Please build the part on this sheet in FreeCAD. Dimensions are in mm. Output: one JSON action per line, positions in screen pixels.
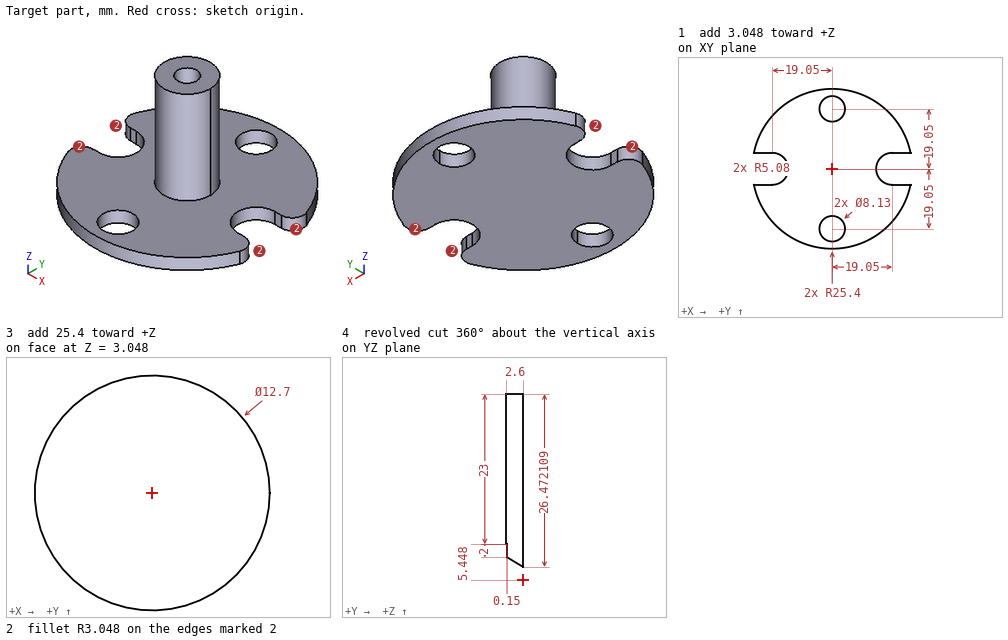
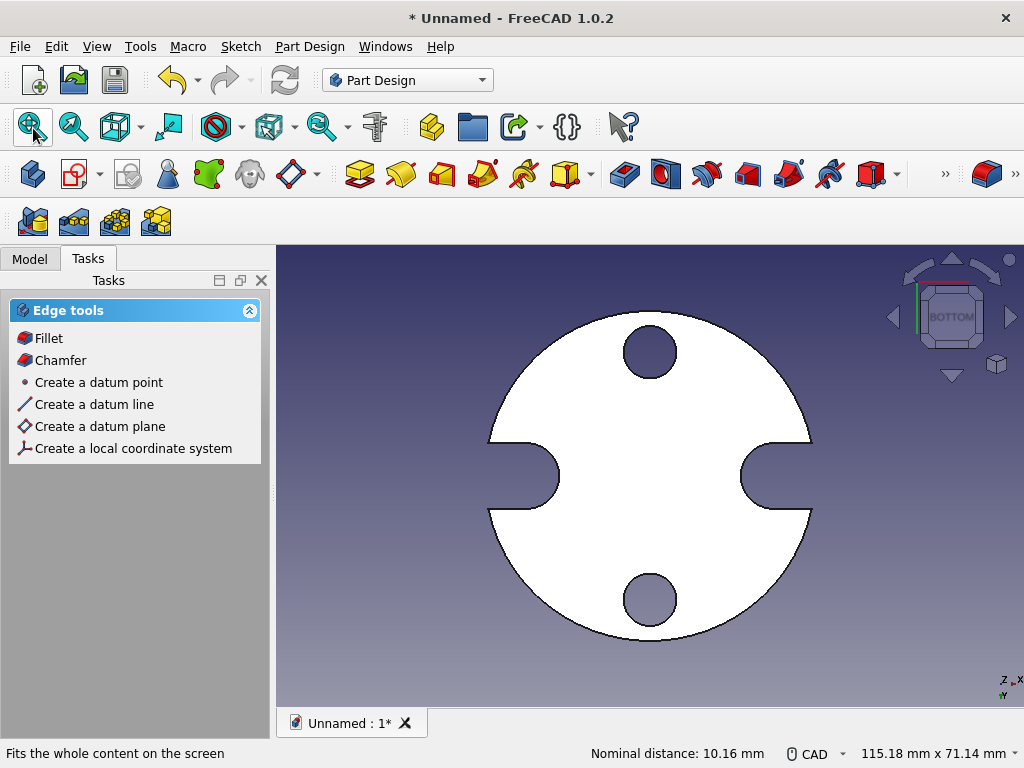
{"action": "key", "text": "4"}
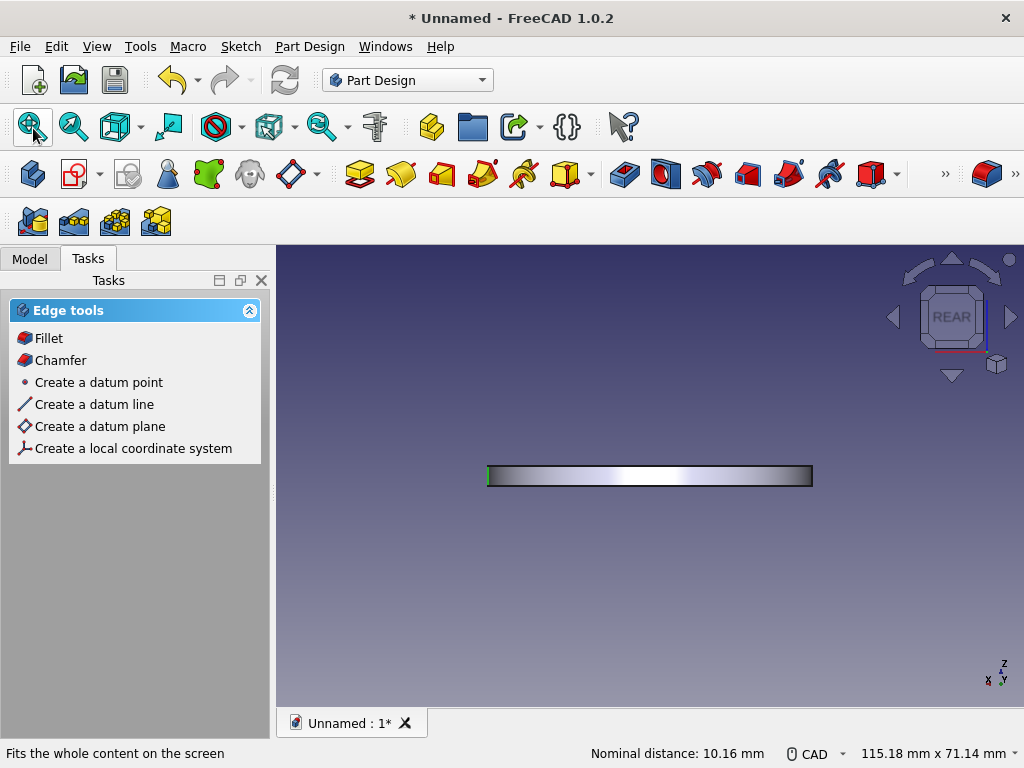
{"action": "left_click", "coordinate": [33, 128]}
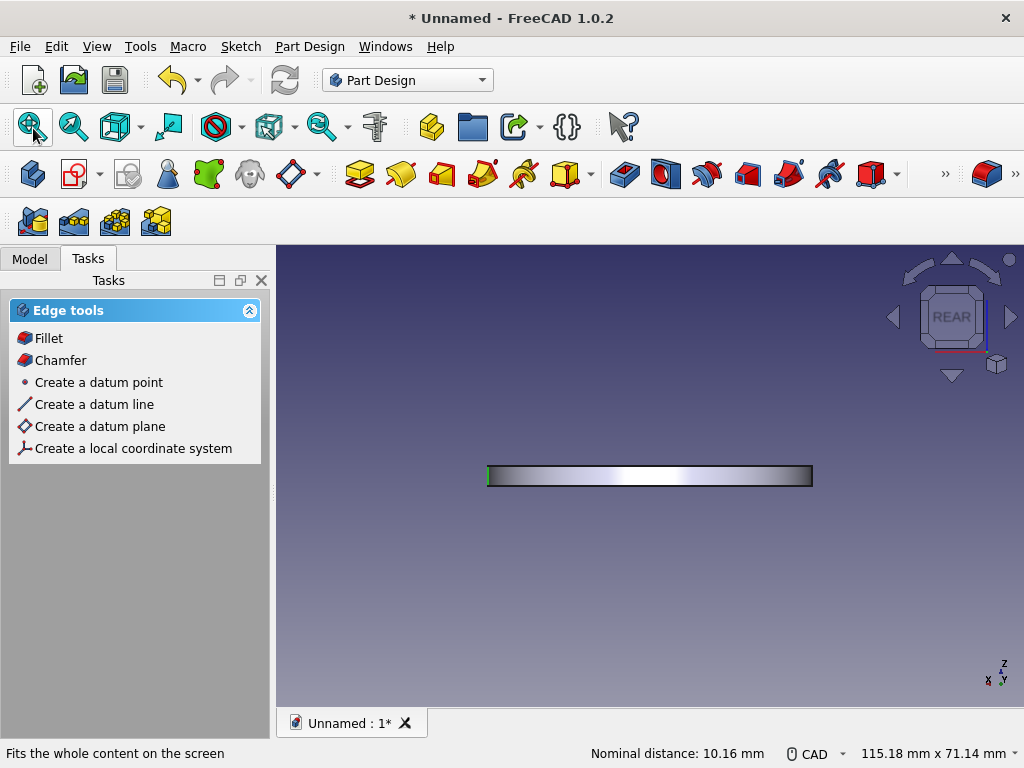
{"action": "scroll", "coordinate": [812, 475], "scroll_direction": "up", "scroll_amount": 4}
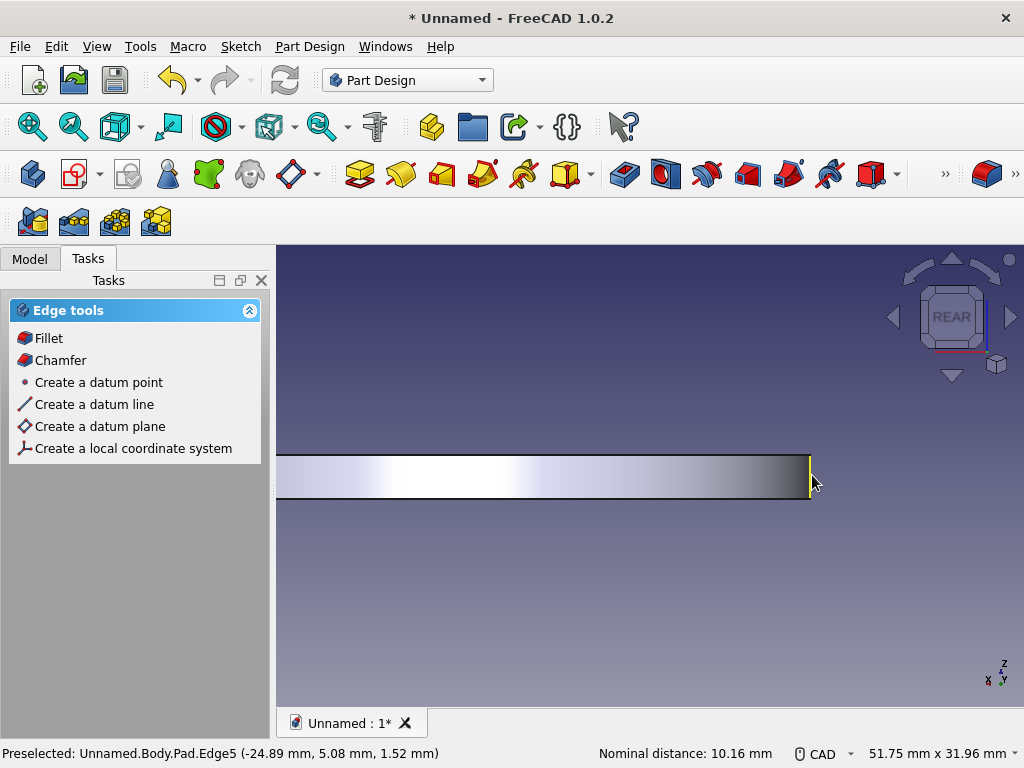
{"action": "left_click", "coordinate": [33, 128]}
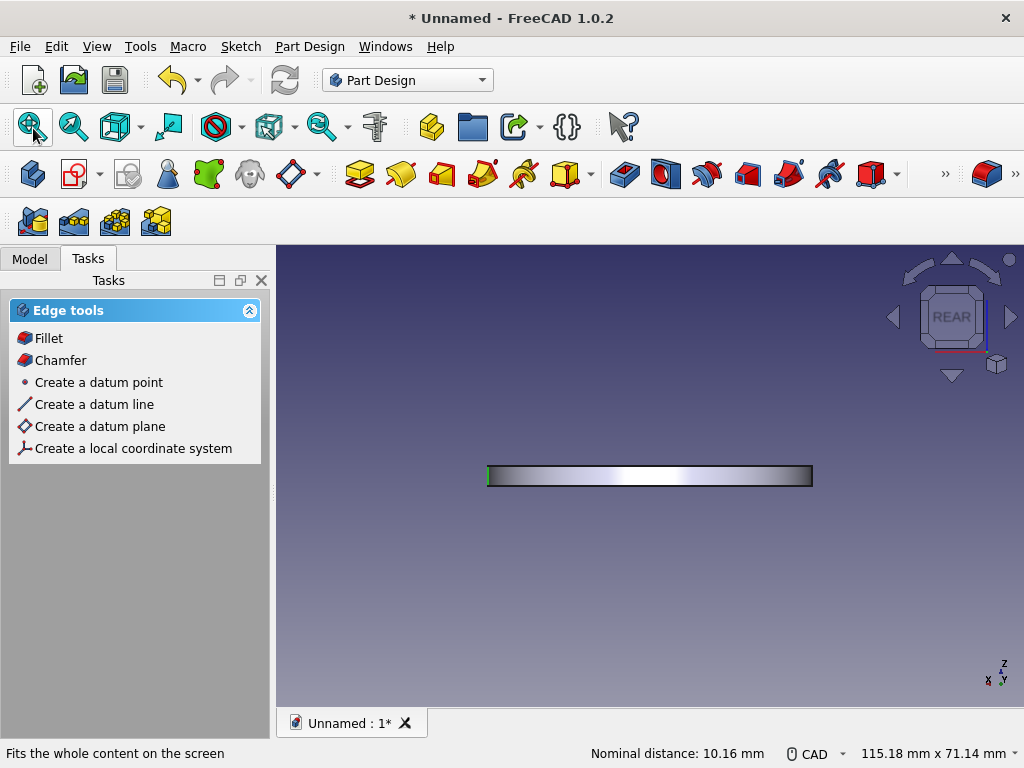
{"action": "key", "text": "6"}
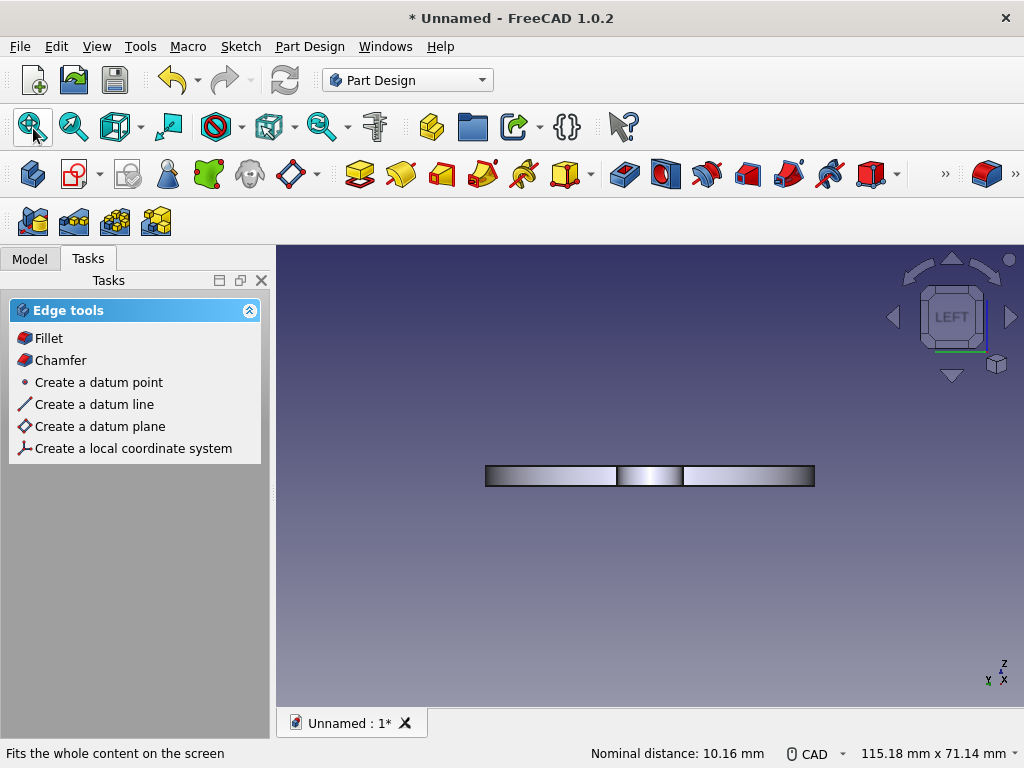
{"action": "left_click", "coordinate": [33, 128]}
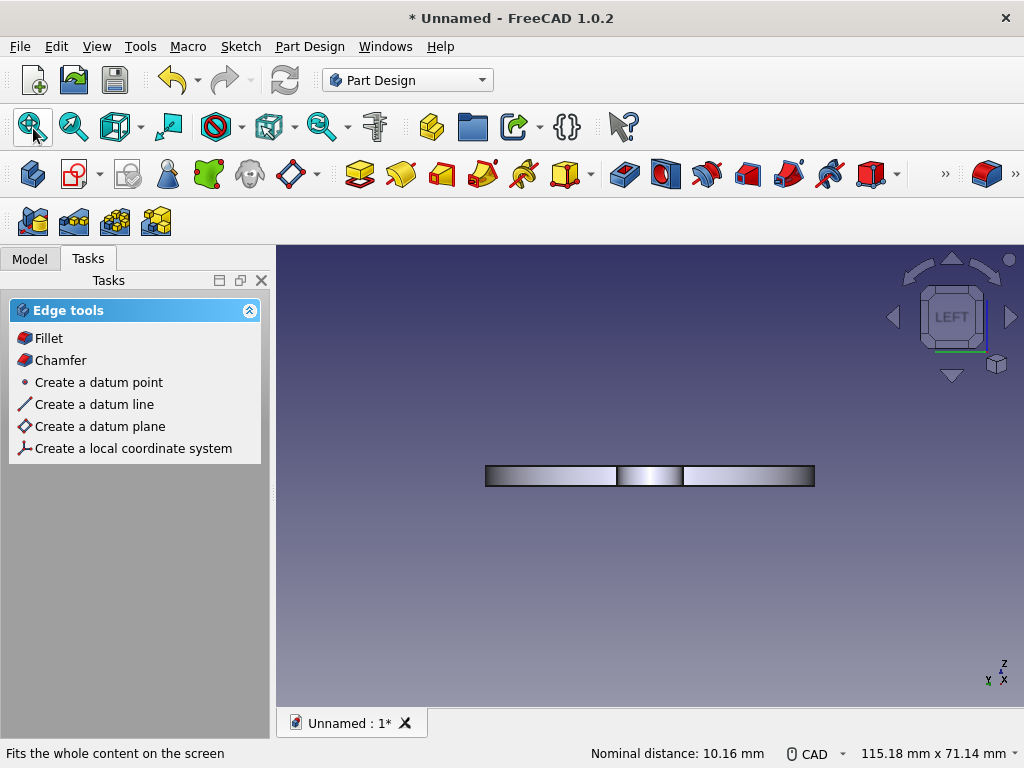
{"action": "left_click", "coordinate": [617, 475], "text": "ctrl"}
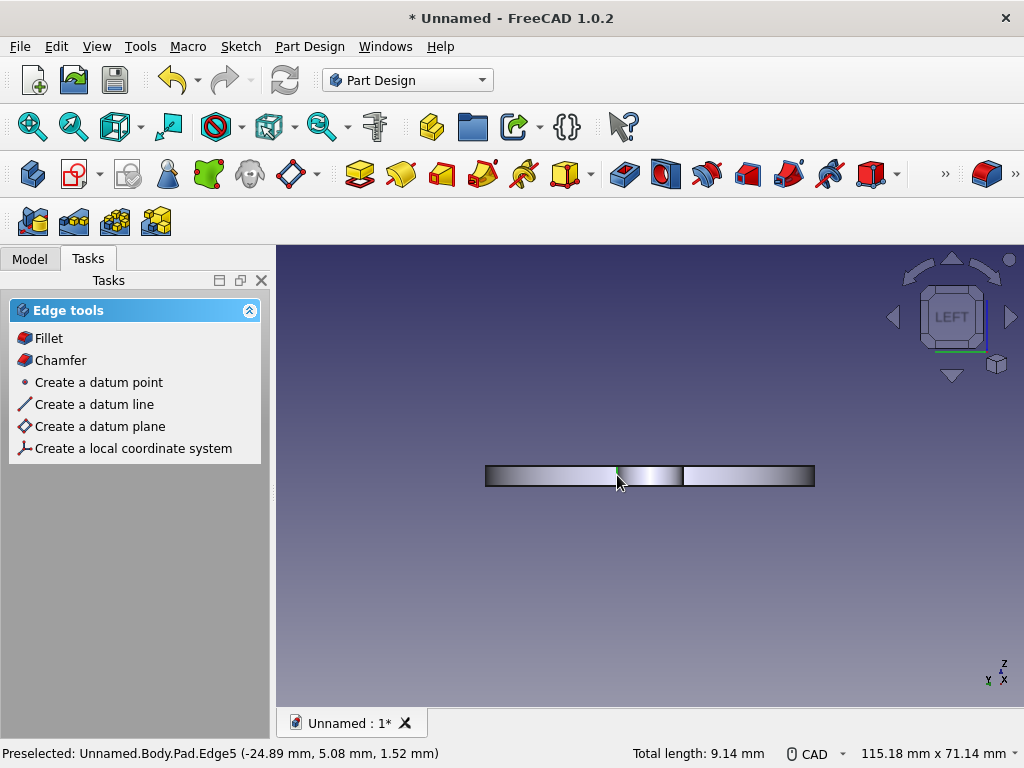
{"action": "left_click", "coordinate": [683, 475], "text": "ctrl"}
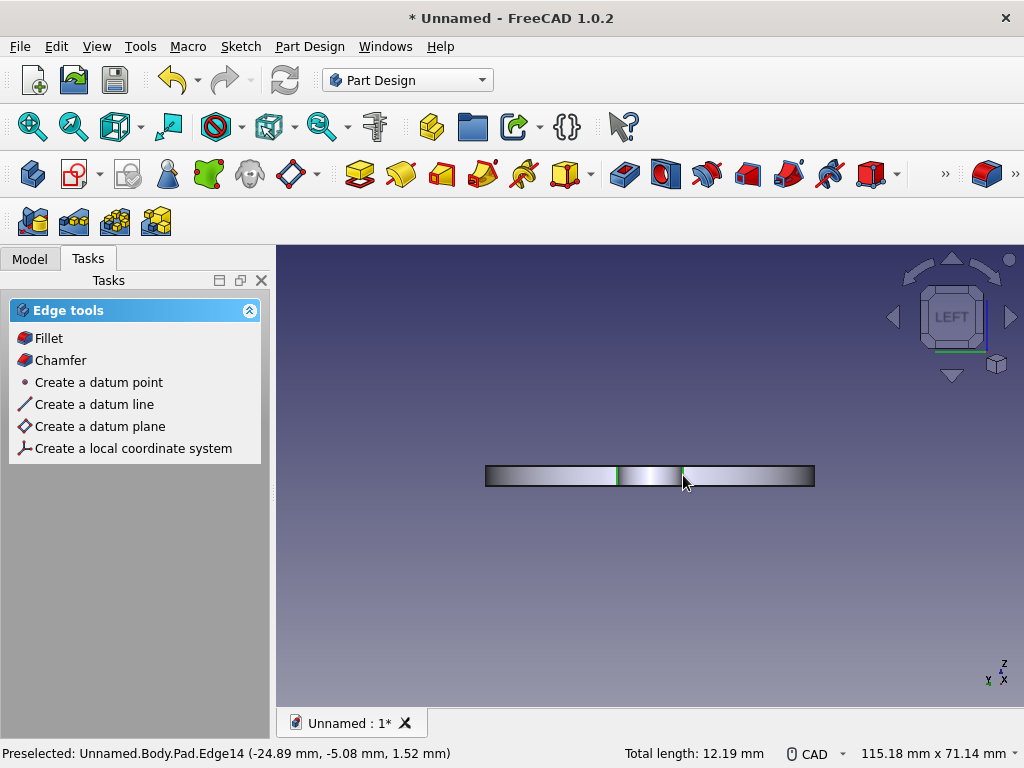
{"action": "left_click", "coordinate": [987, 174]}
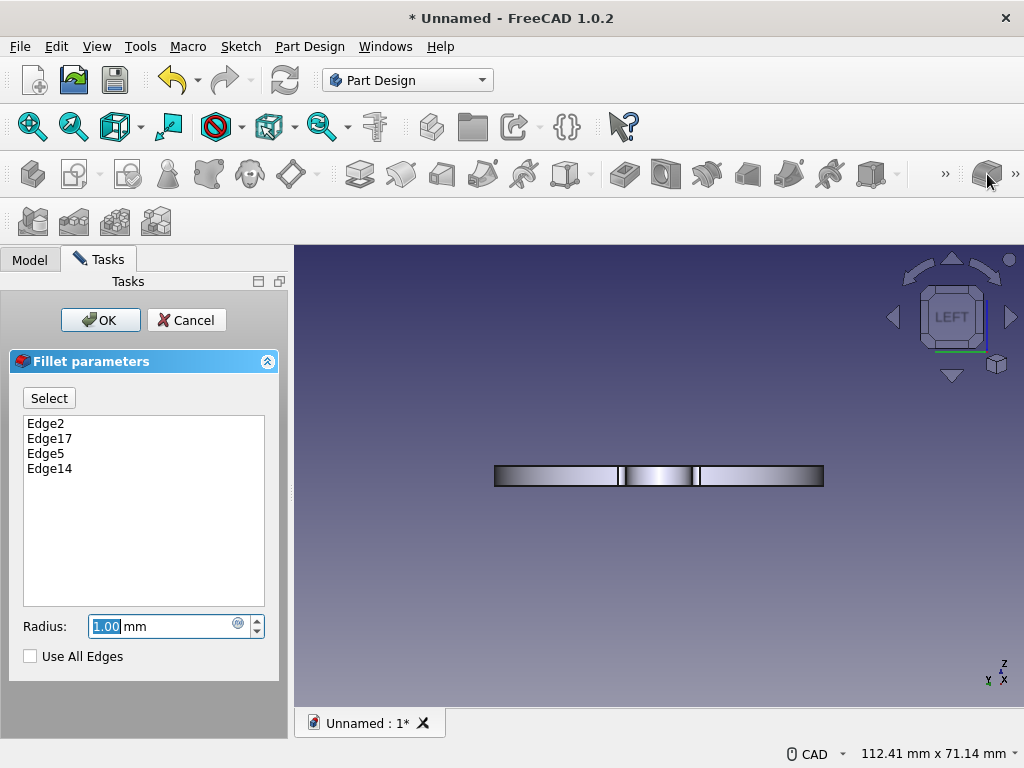
{"action": "type", "text": "3.048"}
{"action": "key", "text": "Tab"}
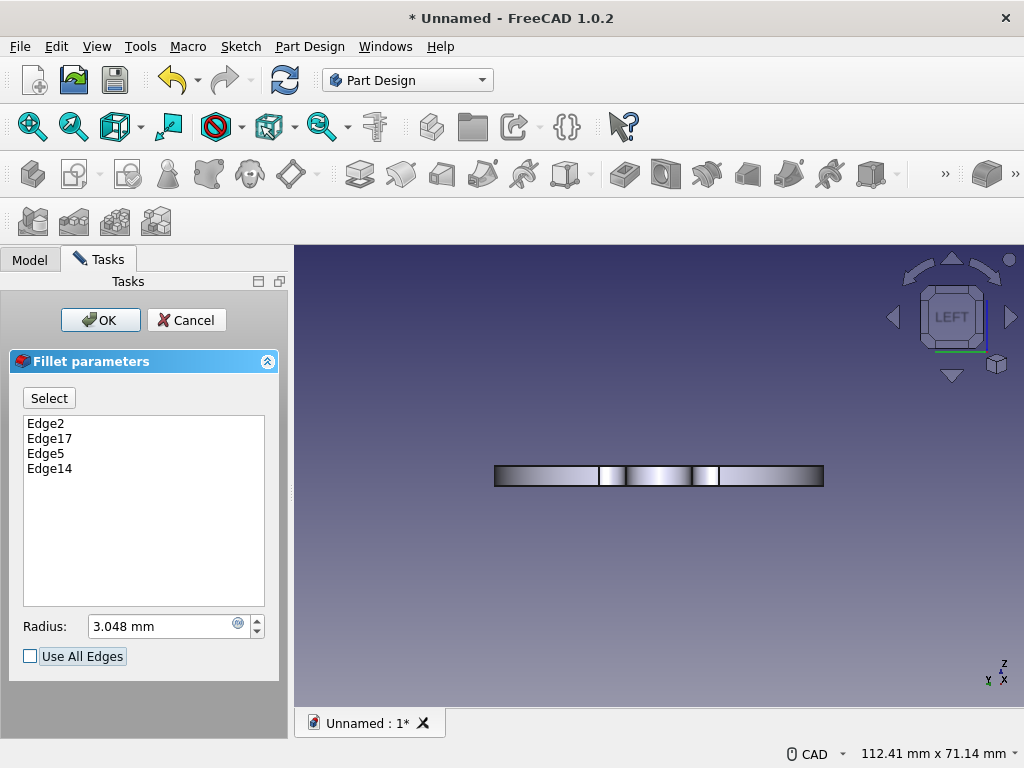
{"action": "left_click", "coordinate": [101, 320]}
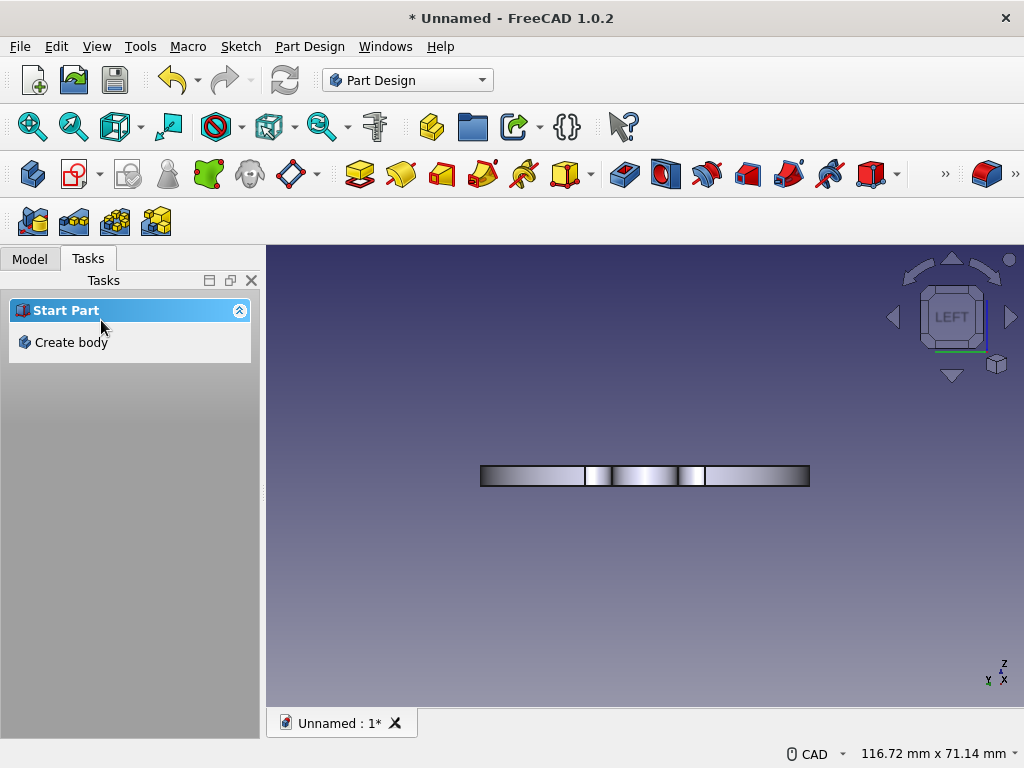
{"action": "left_click", "coordinate": [33, 128]}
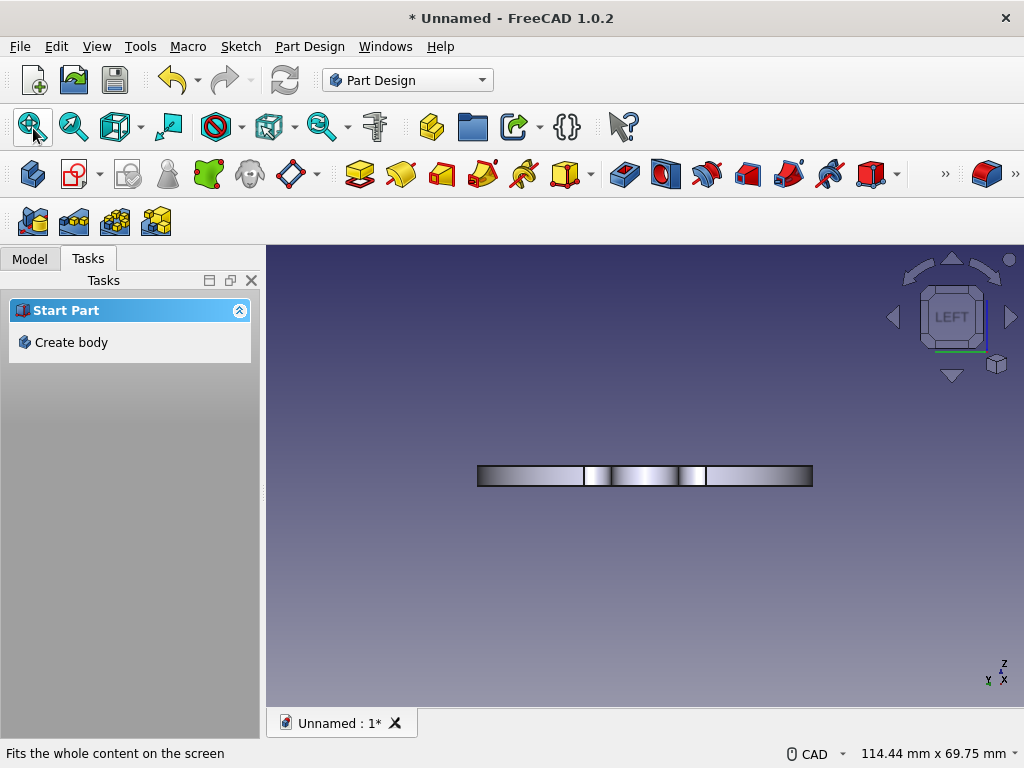
{"action": "key", "text": "0"}